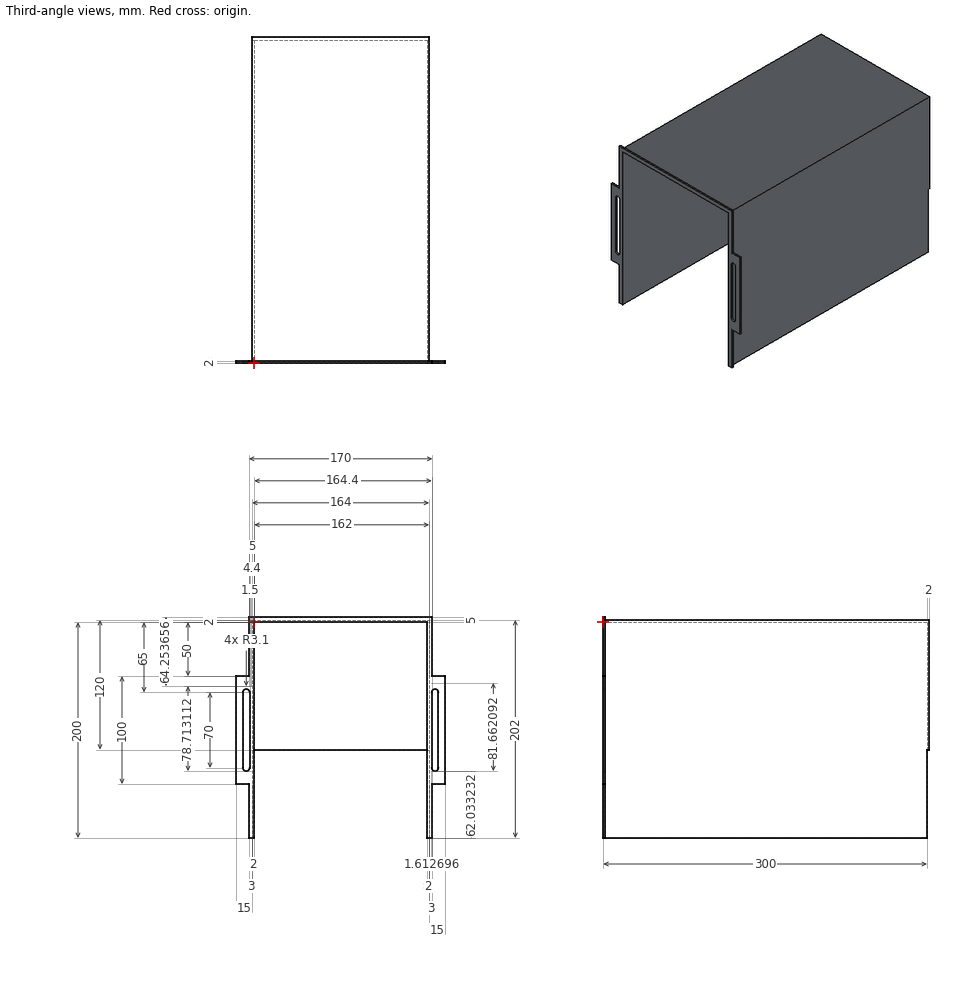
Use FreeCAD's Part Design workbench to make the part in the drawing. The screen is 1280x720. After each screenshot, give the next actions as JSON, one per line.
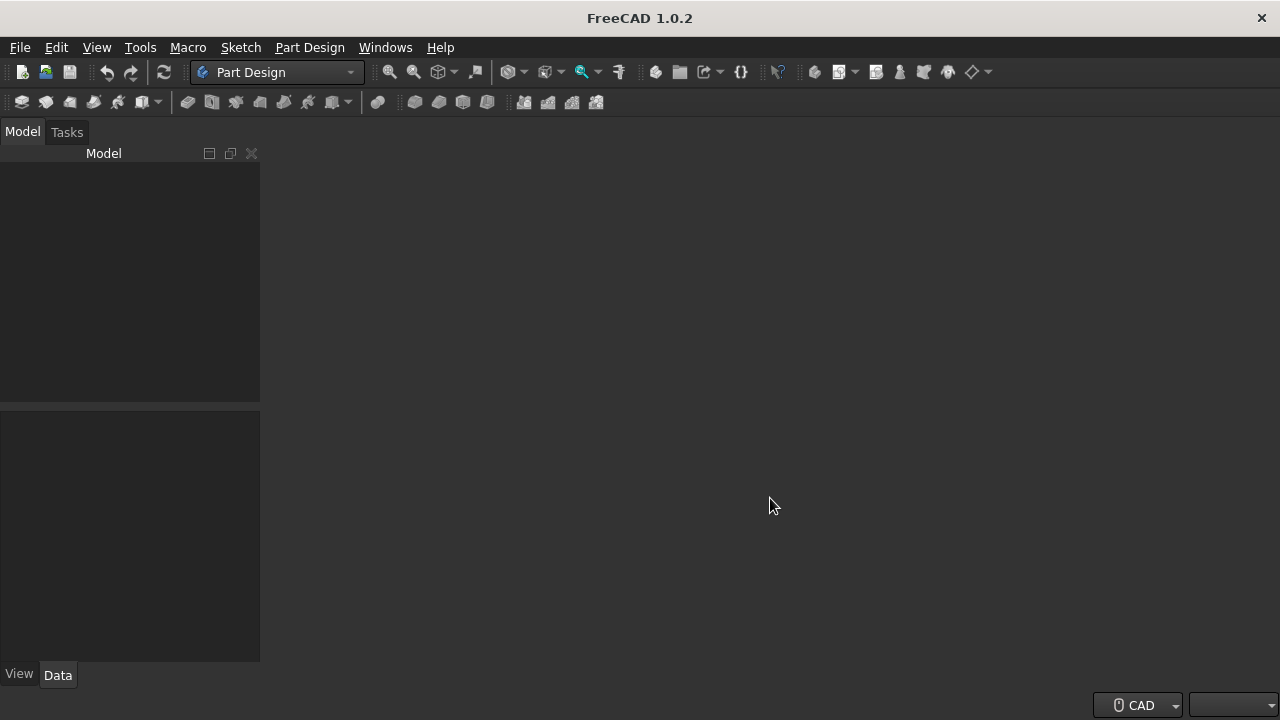
{"action": "left_click", "coordinate": [22, 72]}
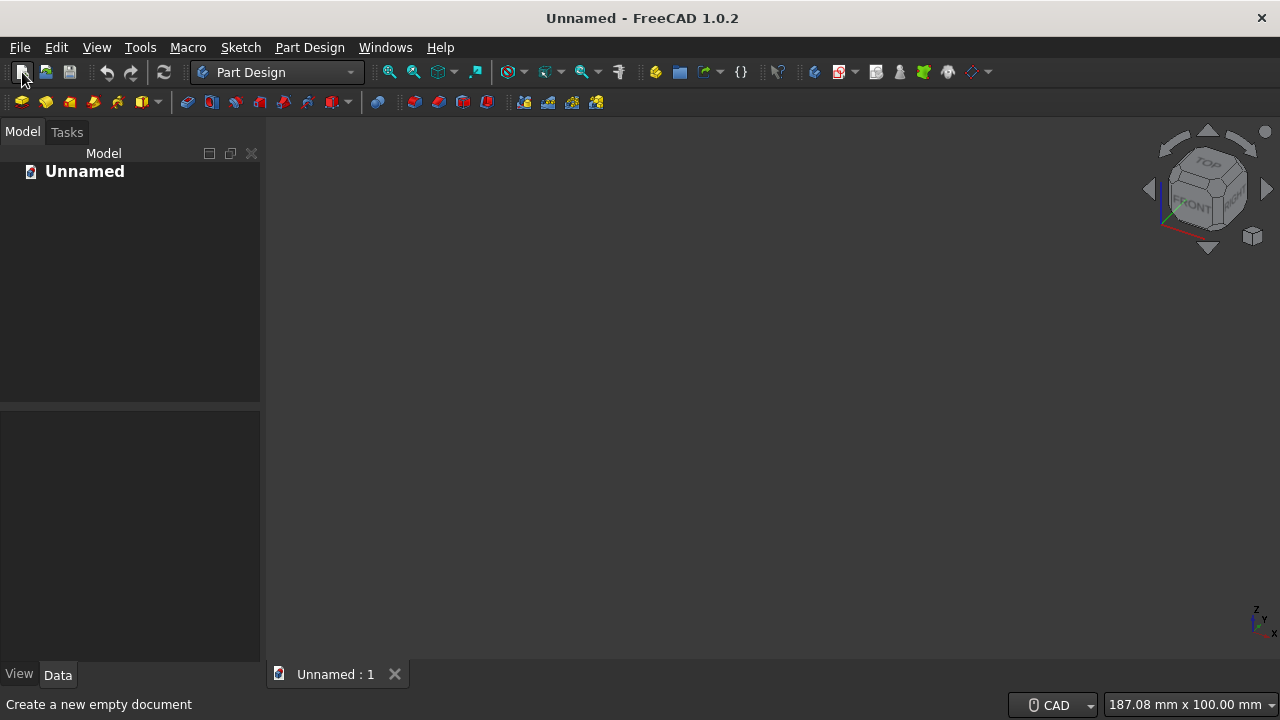
{"action": "left_click", "coordinate": [840, 72]}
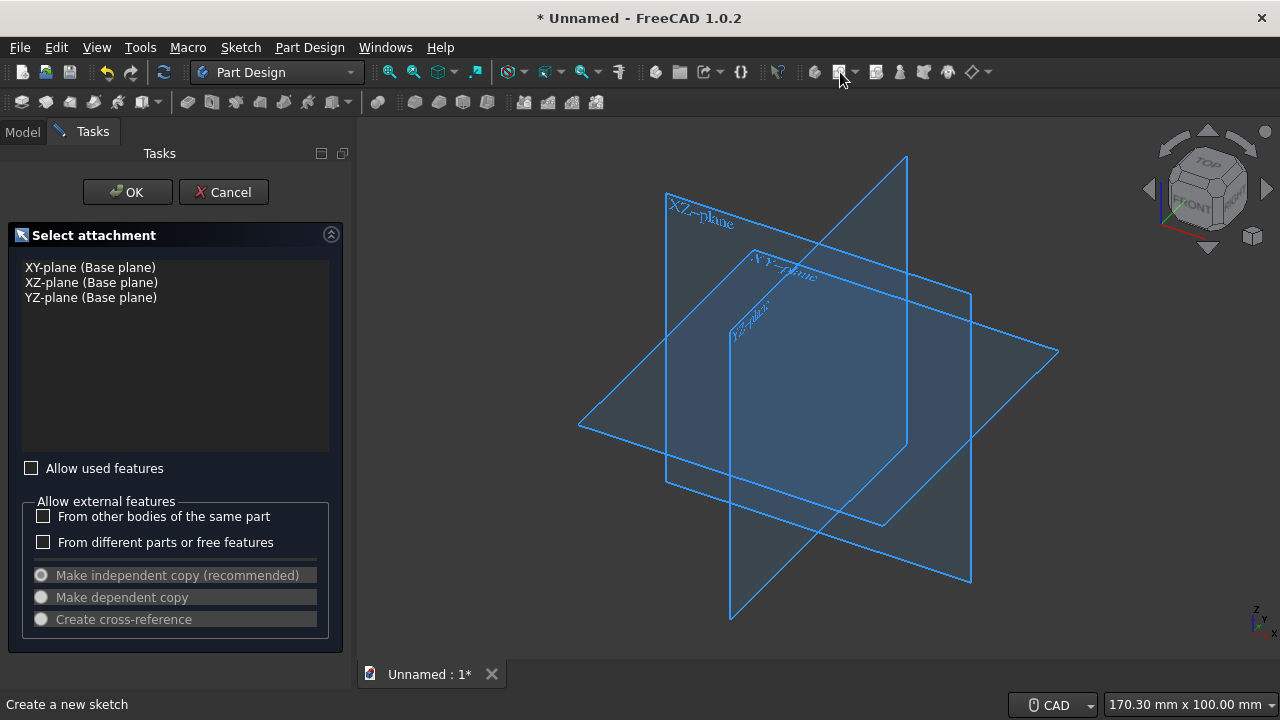
{"action": "left_click", "coordinate": [82, 282]}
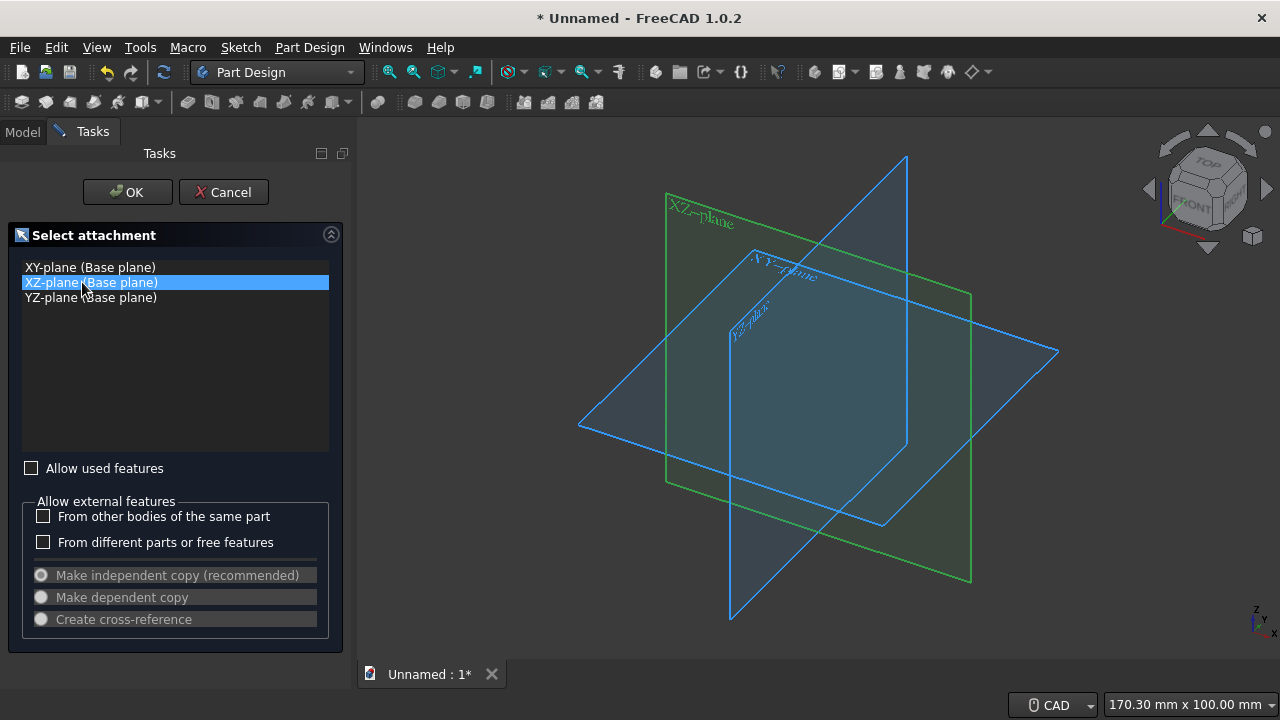
{"action": "left_click", "coordinate": [128, 192]}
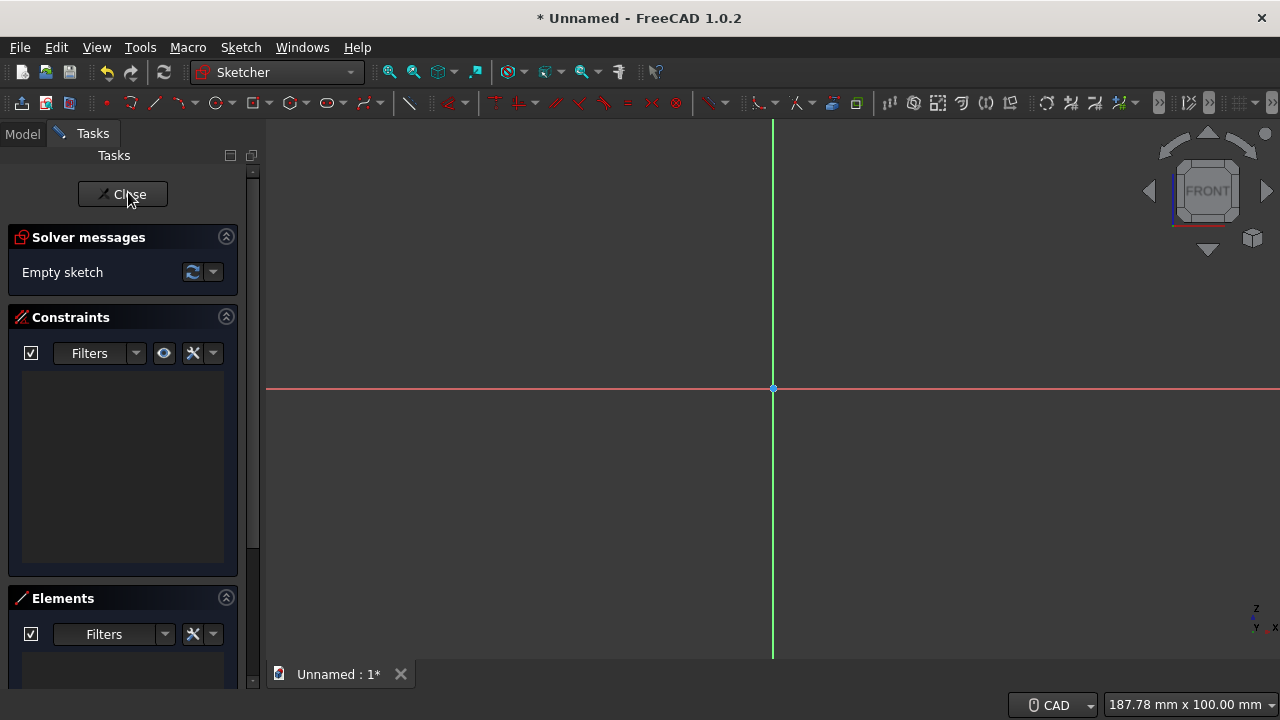
{"action": "scroll", "coordinate": [489, 159], "scroll_direction": "down", "scroll_amount": 6}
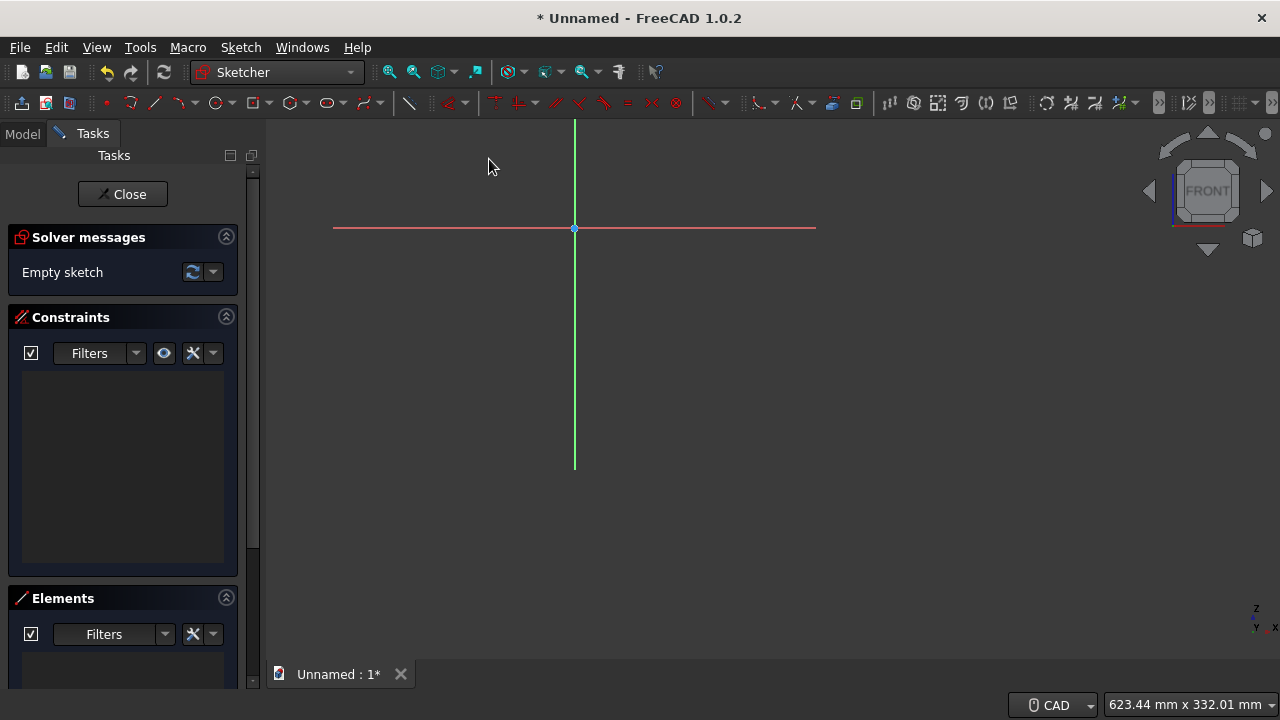
{"action": "left_click", "coordinate": [132, 104]}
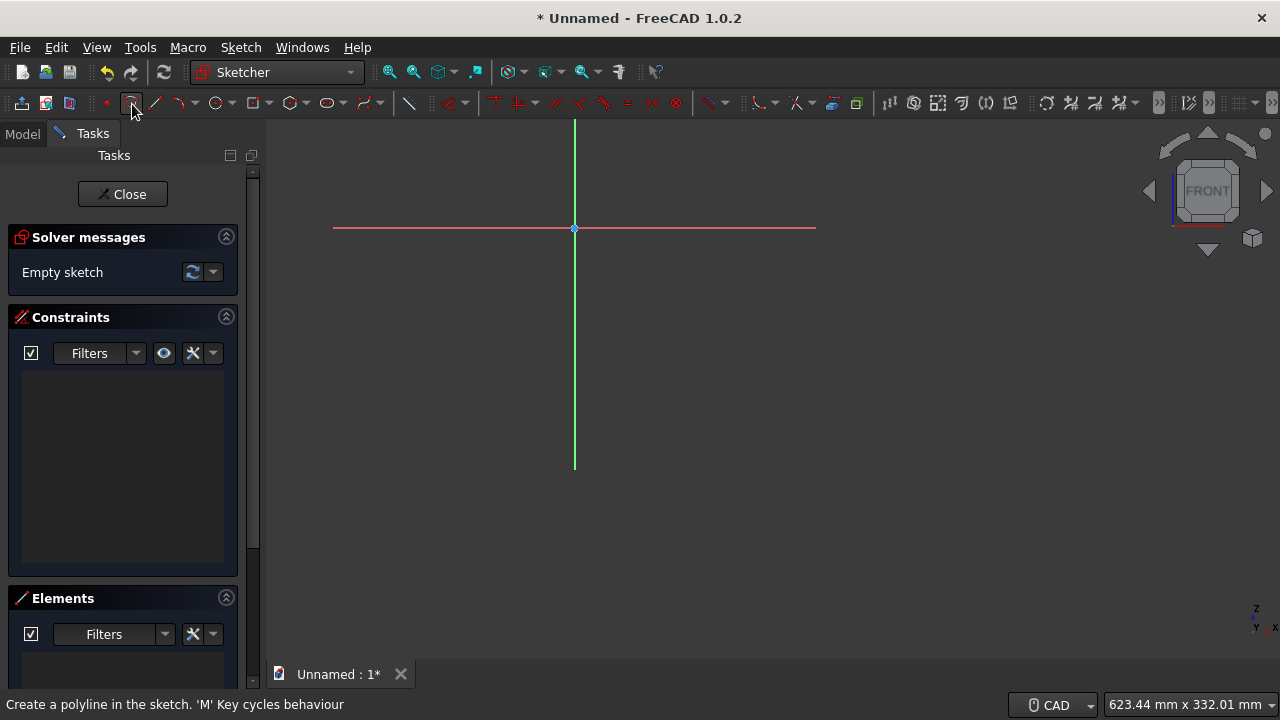
{"action": "left_click", "coordinate": [575, 228]}
{"action": "left_click", "coordinate": [584, 554]}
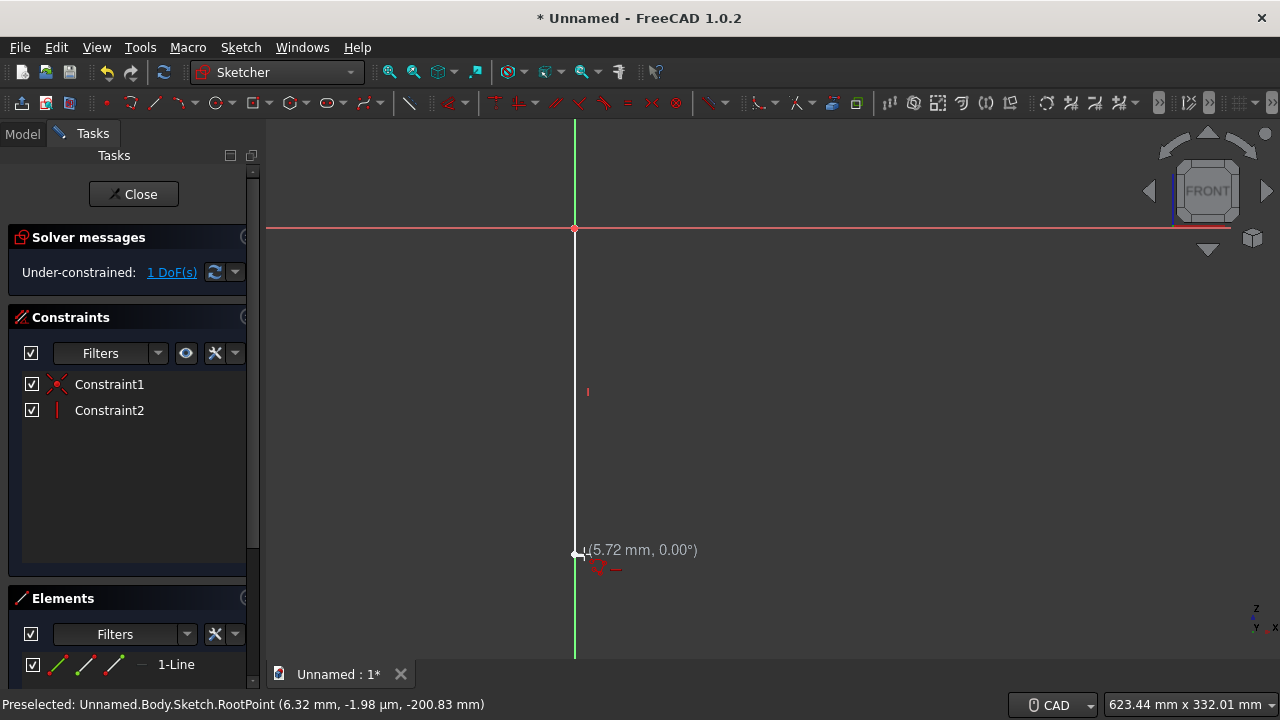
{"action": "scroll", "coordinate": [571, 554], "scroll_direction": "up", "scroll_amount": 8}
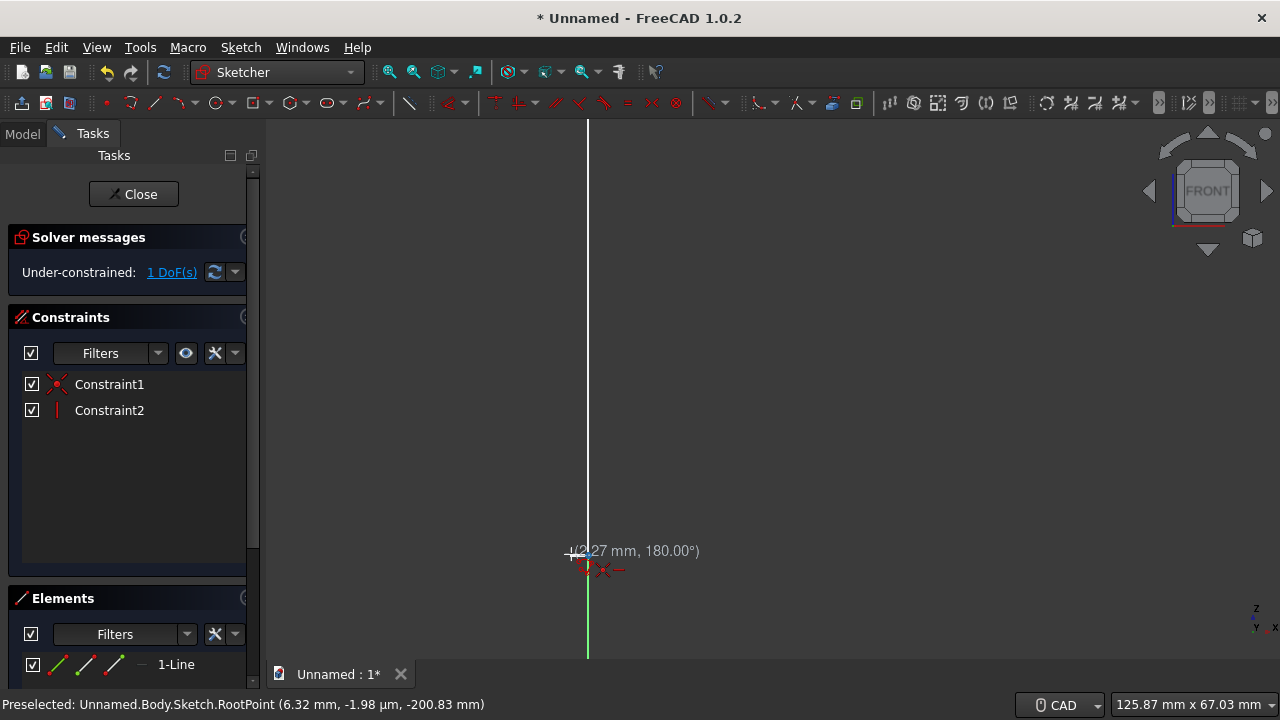
{"action": "left_click", "coordinate": [572, 551]}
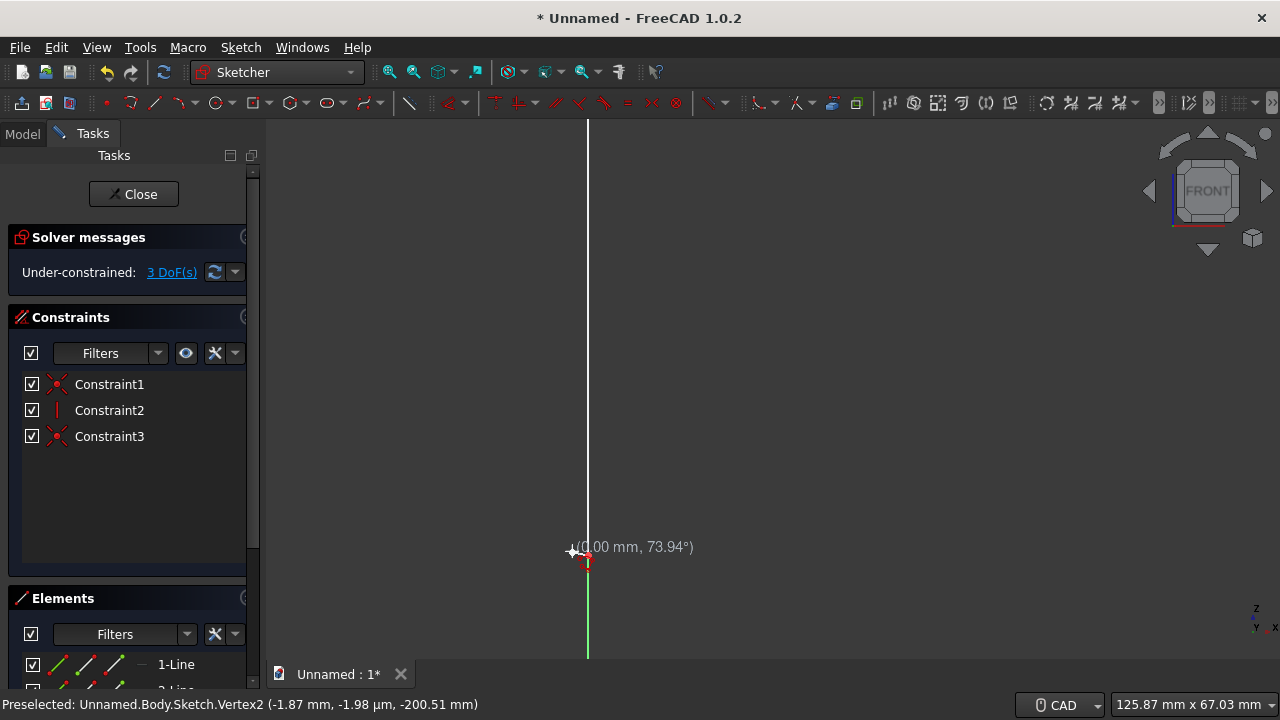
{"action": "scroll", "coordinate": [571, 554], "scroll_direction": "down", "scroll_amount": 8}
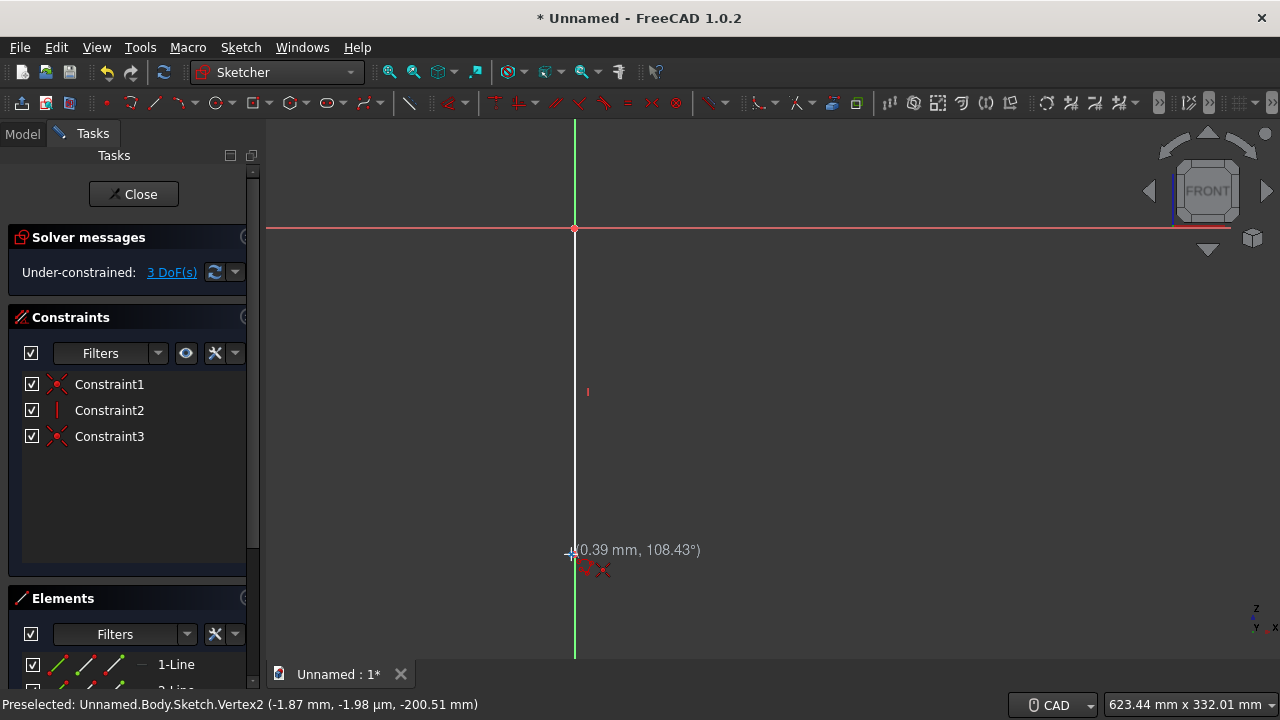
{"action": "scroll", "coordinate": [571, 225], "scroll_direction": "up", "scroll_amount": 8}